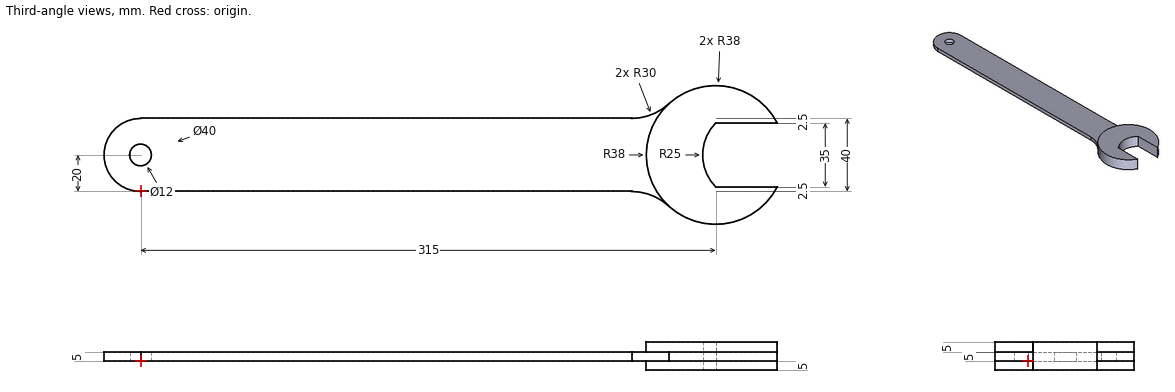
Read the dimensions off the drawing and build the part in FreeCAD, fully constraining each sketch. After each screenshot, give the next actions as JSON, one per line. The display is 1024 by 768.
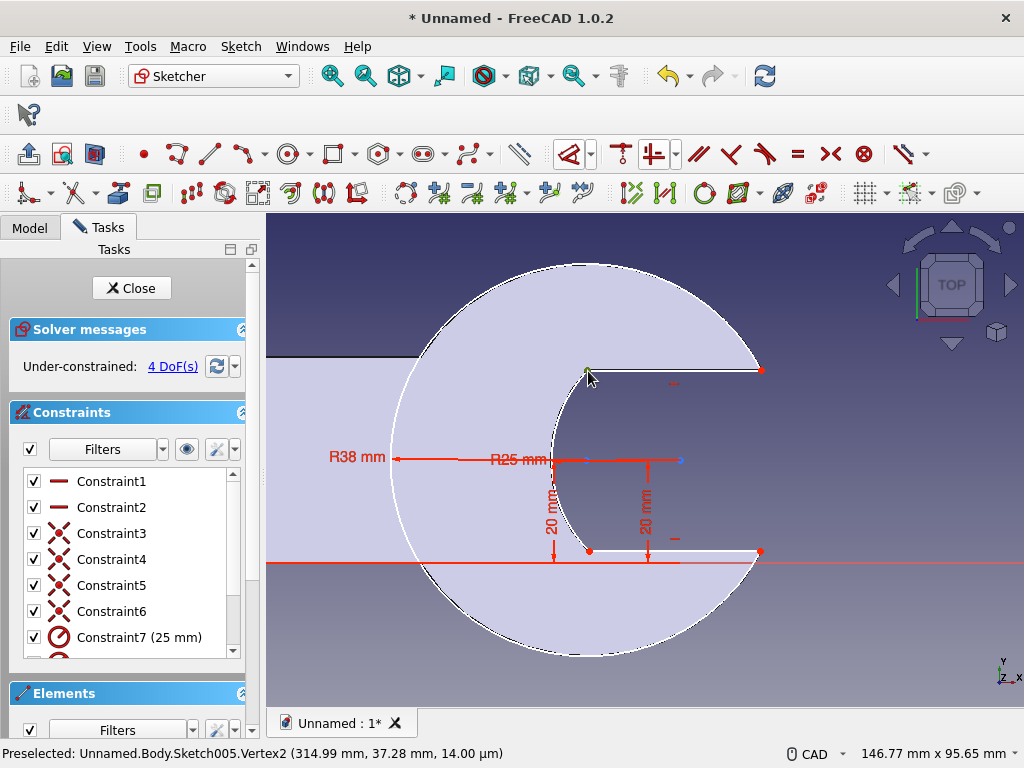
{"action": "key", "text": "l"}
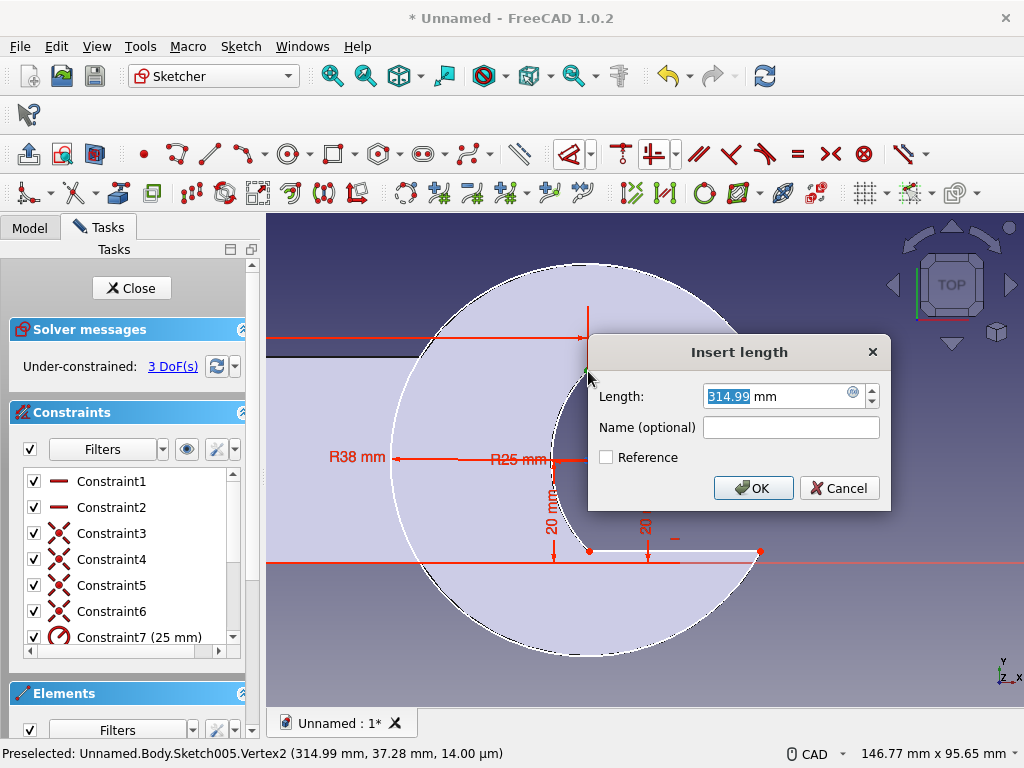
{"action": "type", "text": "315"}
{"action": "key", "text": "Return"}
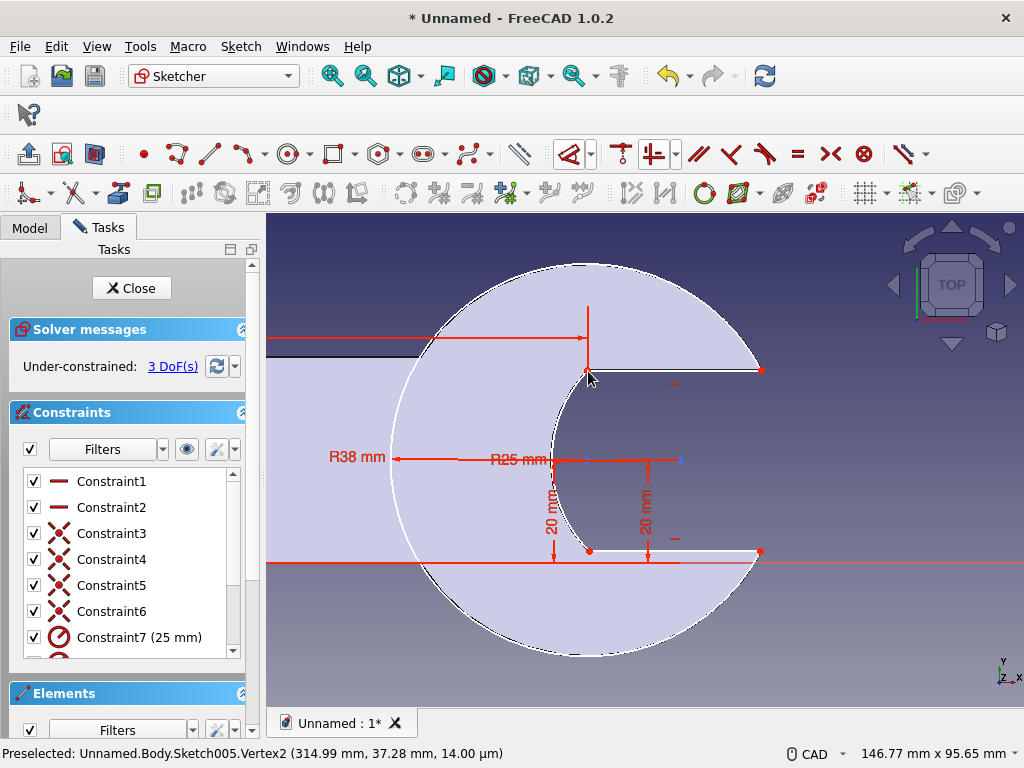
{"action": "left_click", "coordinate": [589, 551]}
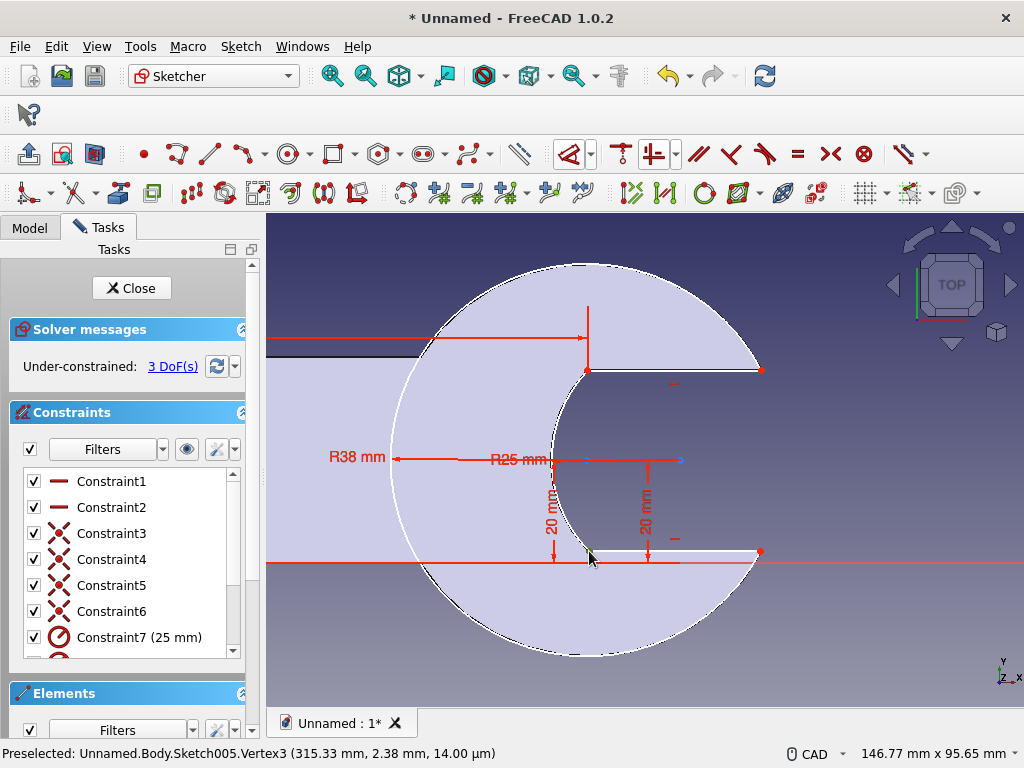
{"action": "left_click", "coordinate": [590, 154]}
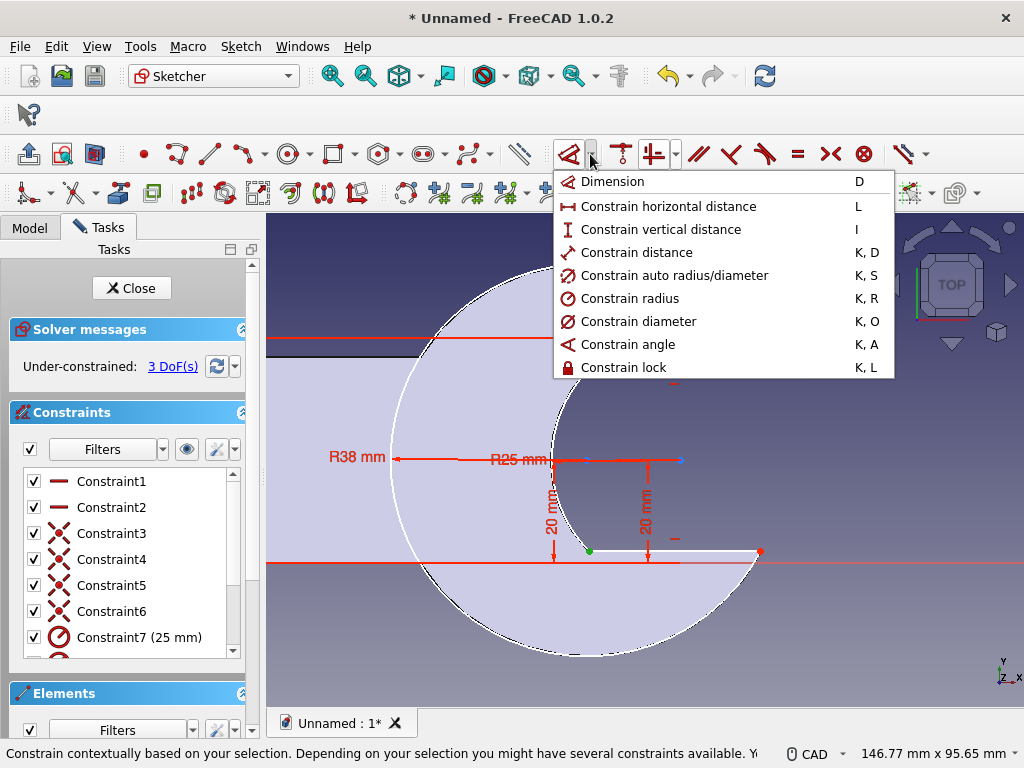
{"action": "left_click", "coordinate": [724, 206]}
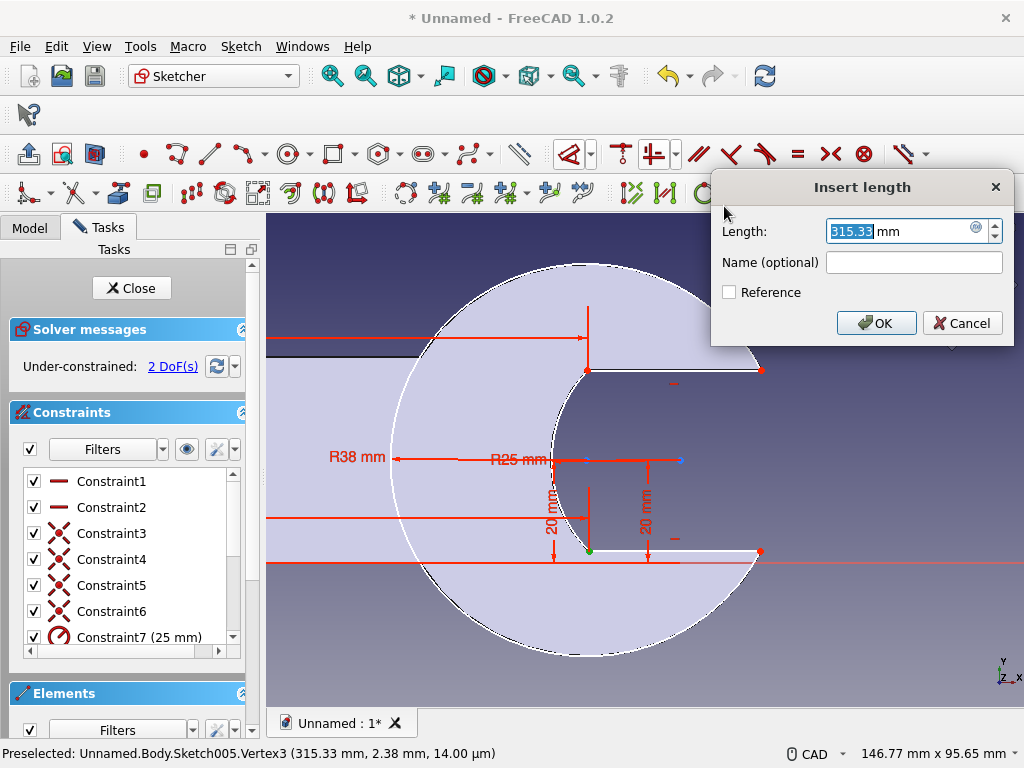
{"action": "type", "text": "315"}
{"action": "key", "text": "Return"}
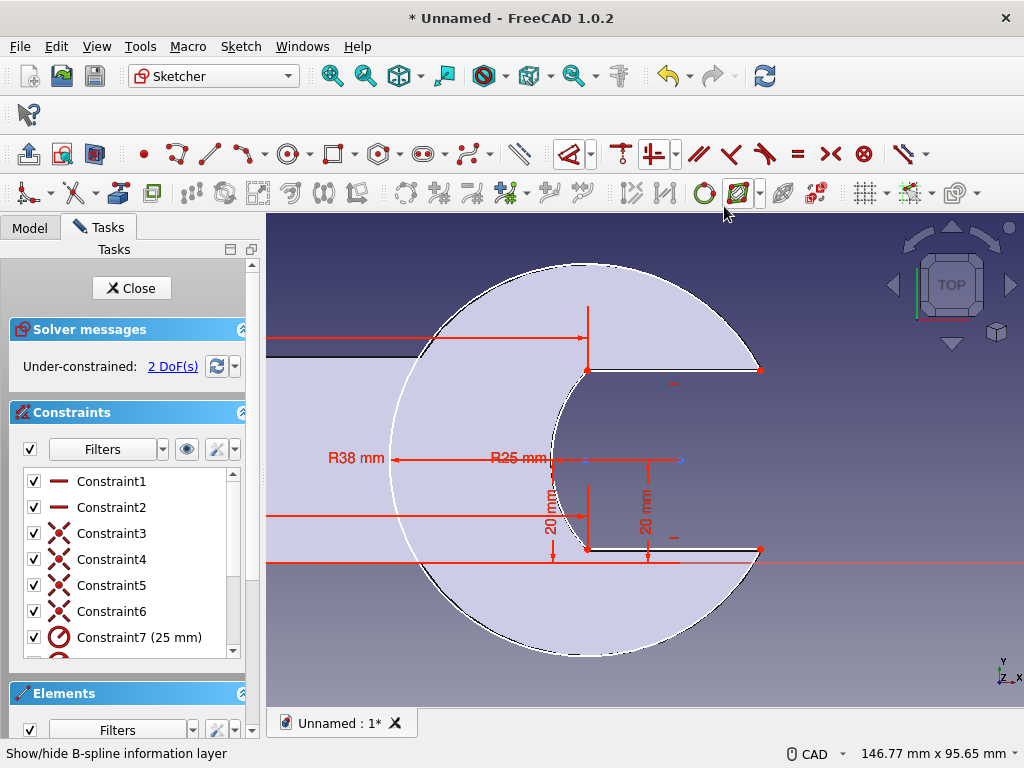
{"action": "scroll", "coordinate": [588, 549], "scroll_direction": "up", "scroll_amount": 6}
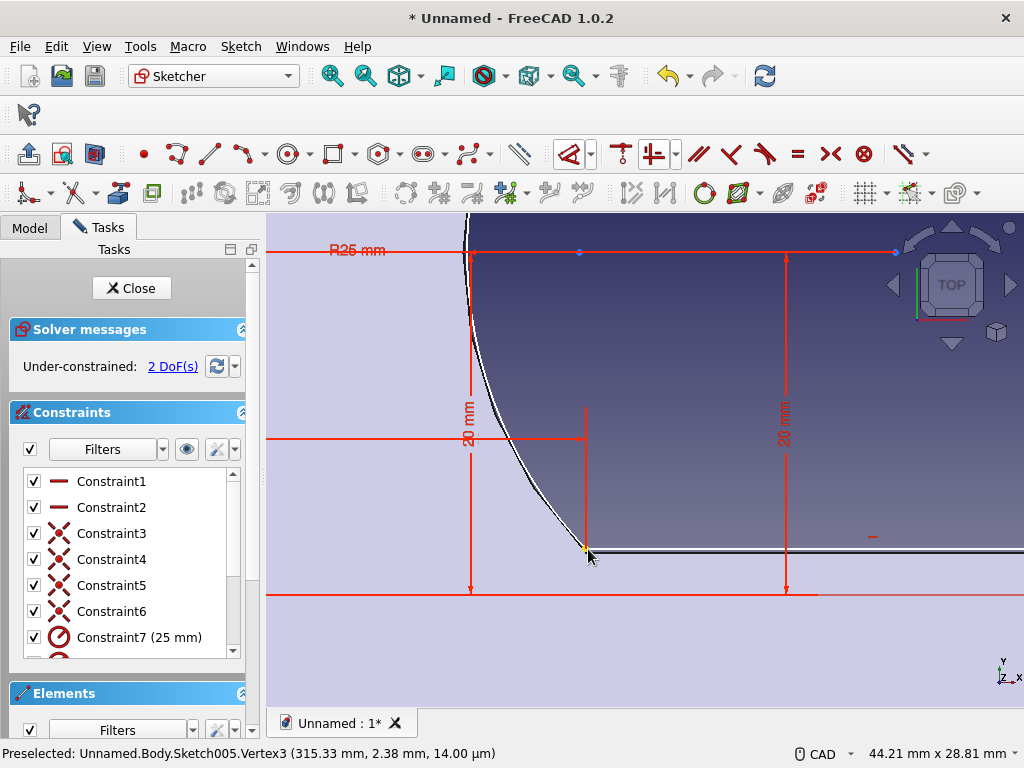
{"action": "left_click", "coordinate": [586, 549]}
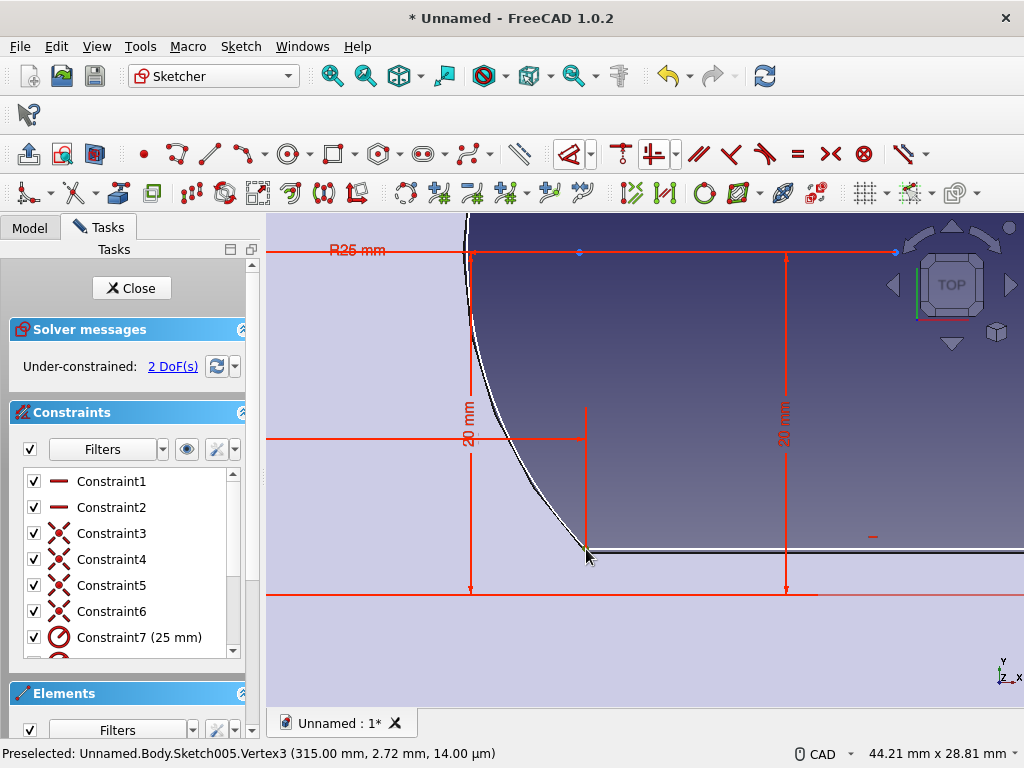
{"action": "left_click", "coordinate": [590, 154]}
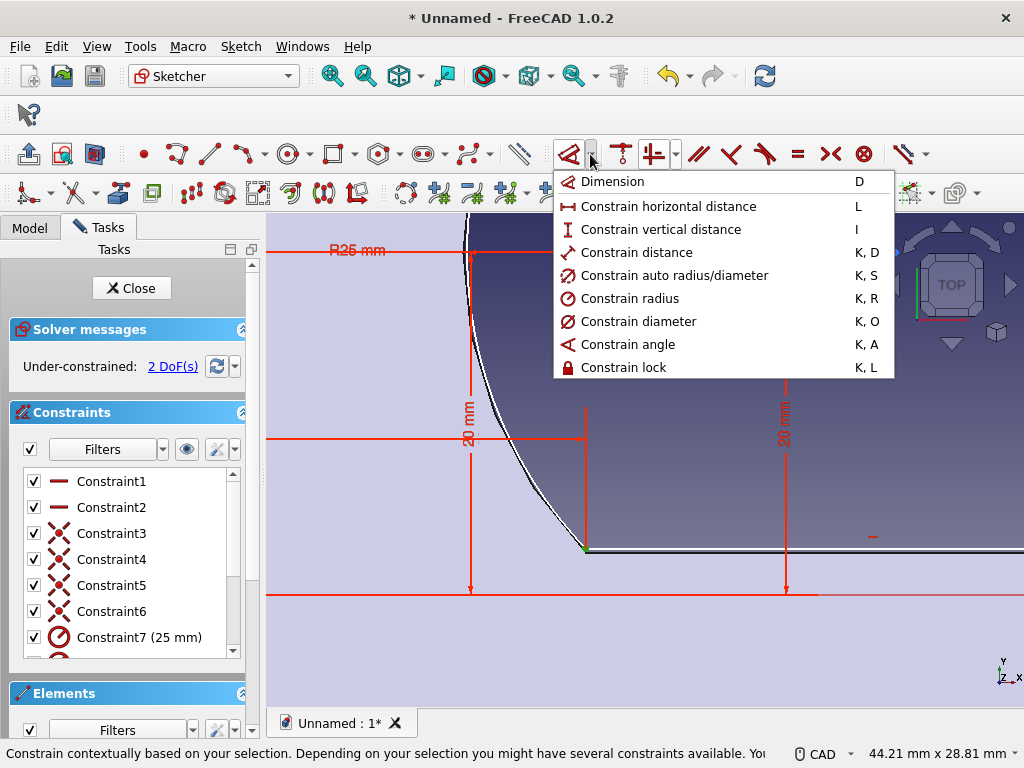
{"action": "left_click", "coordinate": [724, 230]}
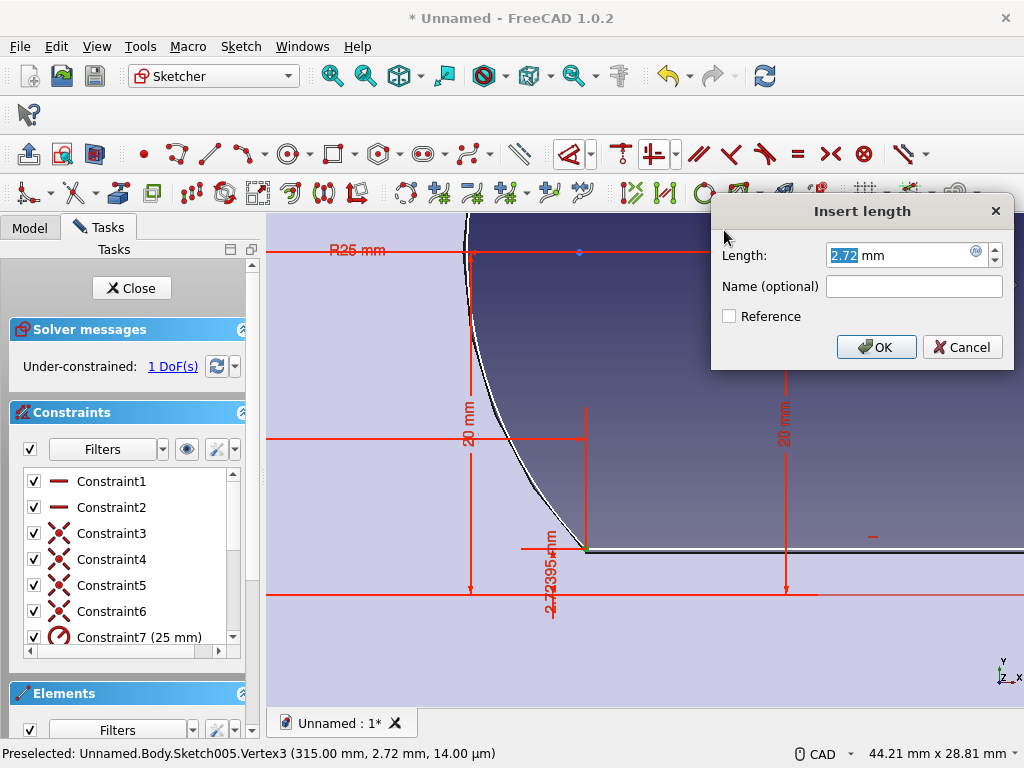
{"action": "type", "text": "2.5"}
{"action": "key", "text": "Return"}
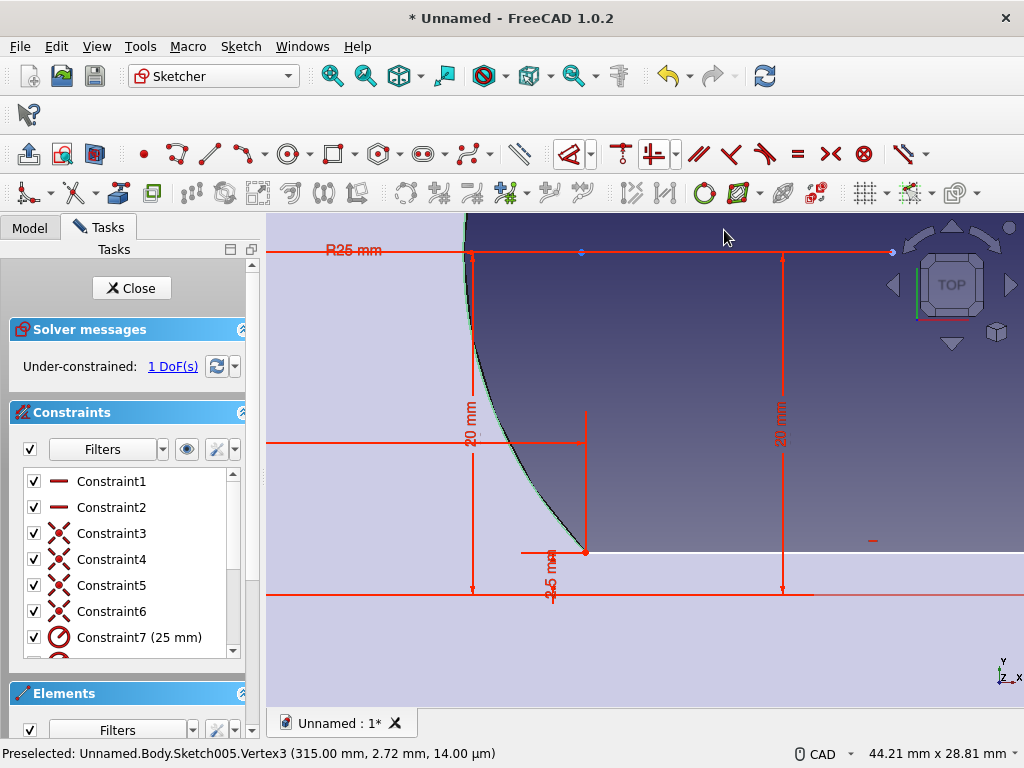
{"action": "left_click", "coordinate": [582, 252]}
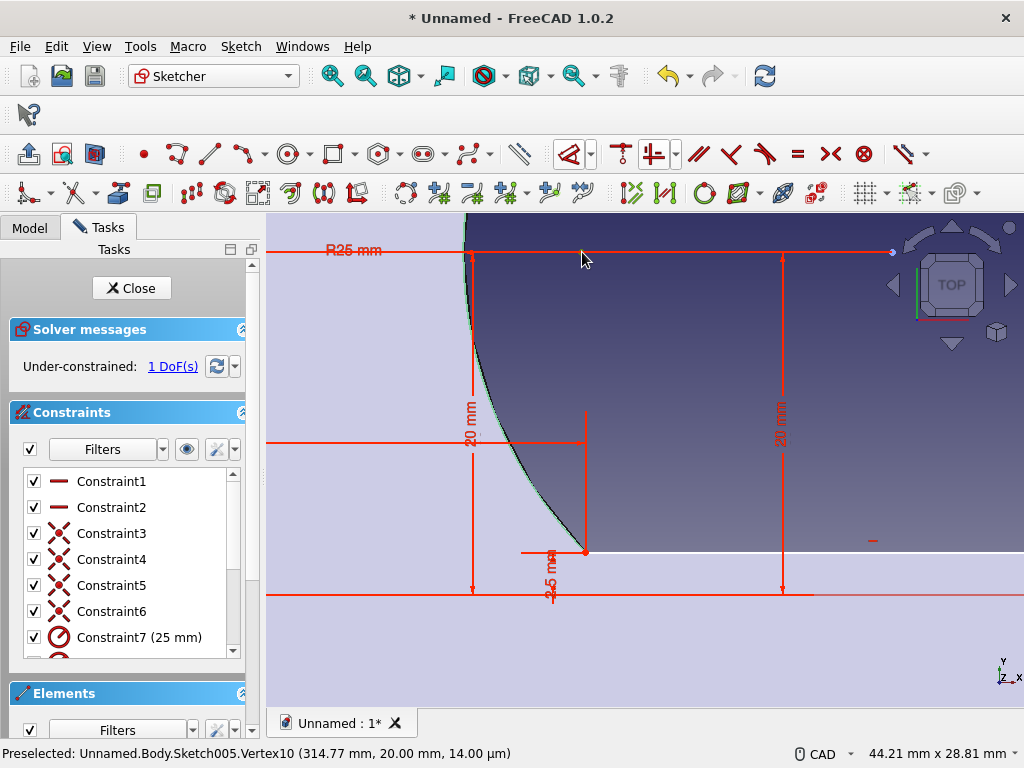
{"action": "key", "text": "l"}